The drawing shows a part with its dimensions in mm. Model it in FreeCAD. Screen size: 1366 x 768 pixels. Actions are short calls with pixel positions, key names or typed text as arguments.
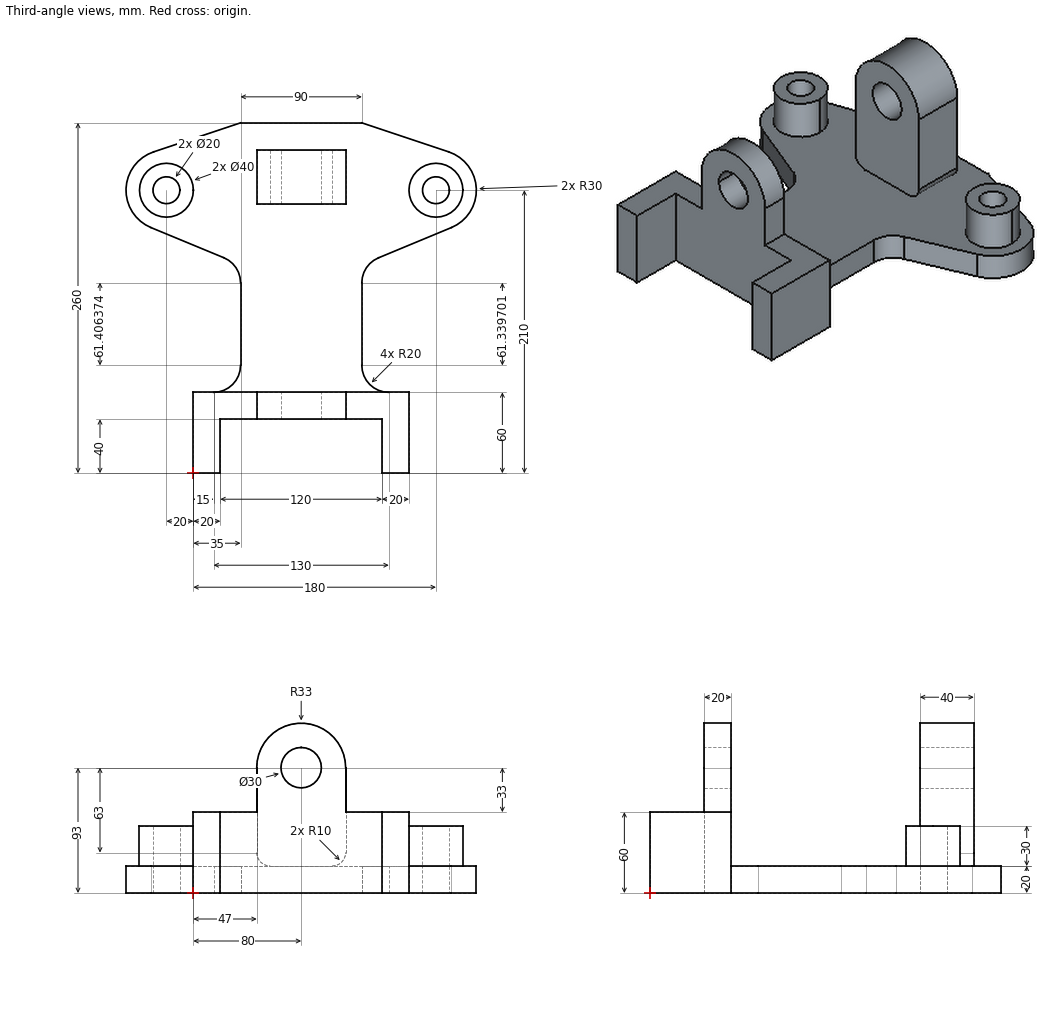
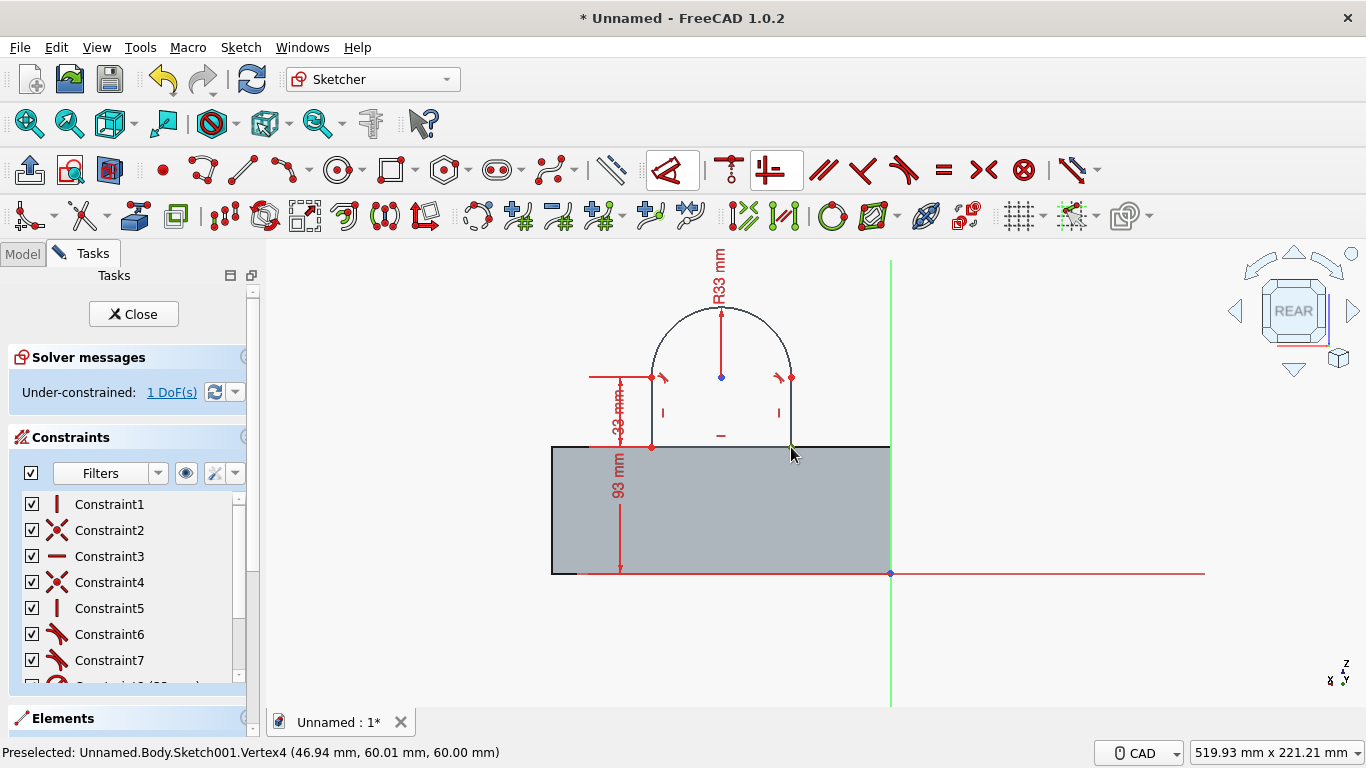
key(l)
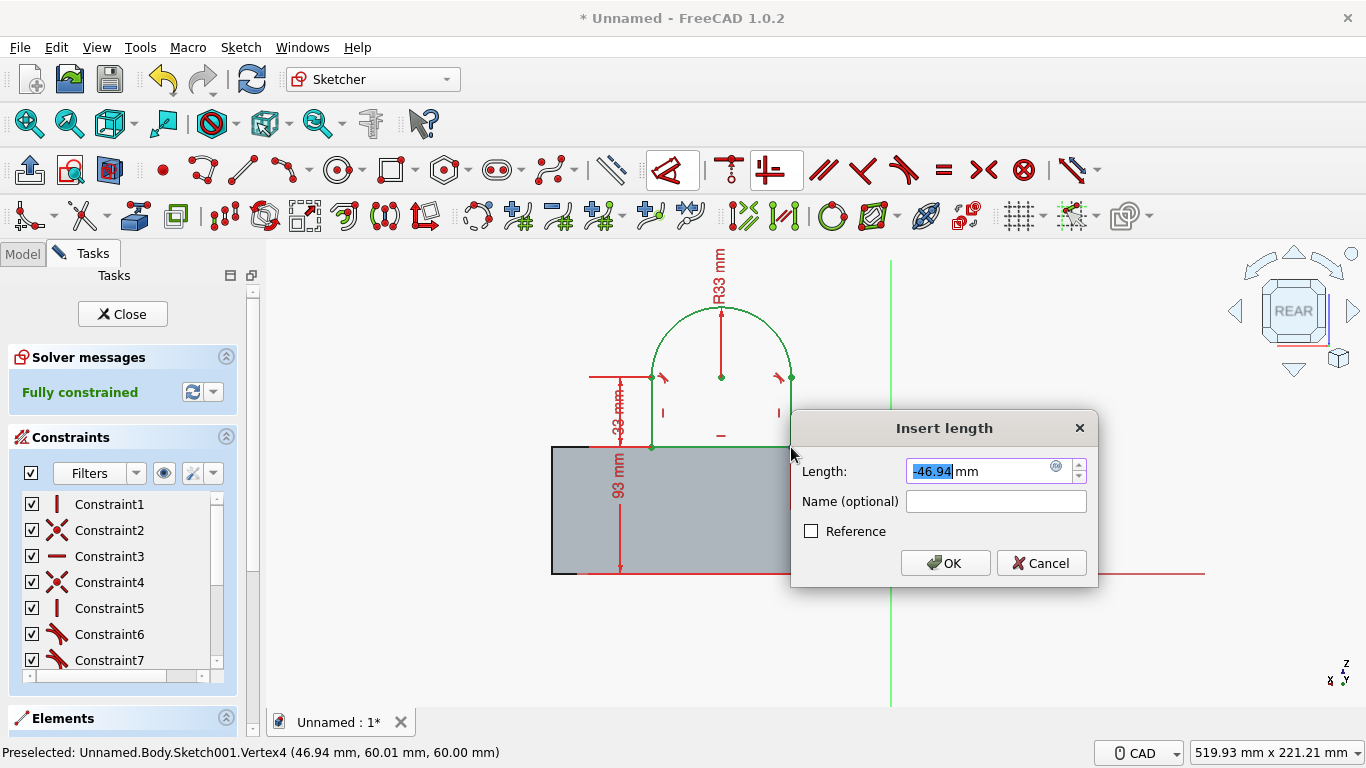
text(-47)
key(Return)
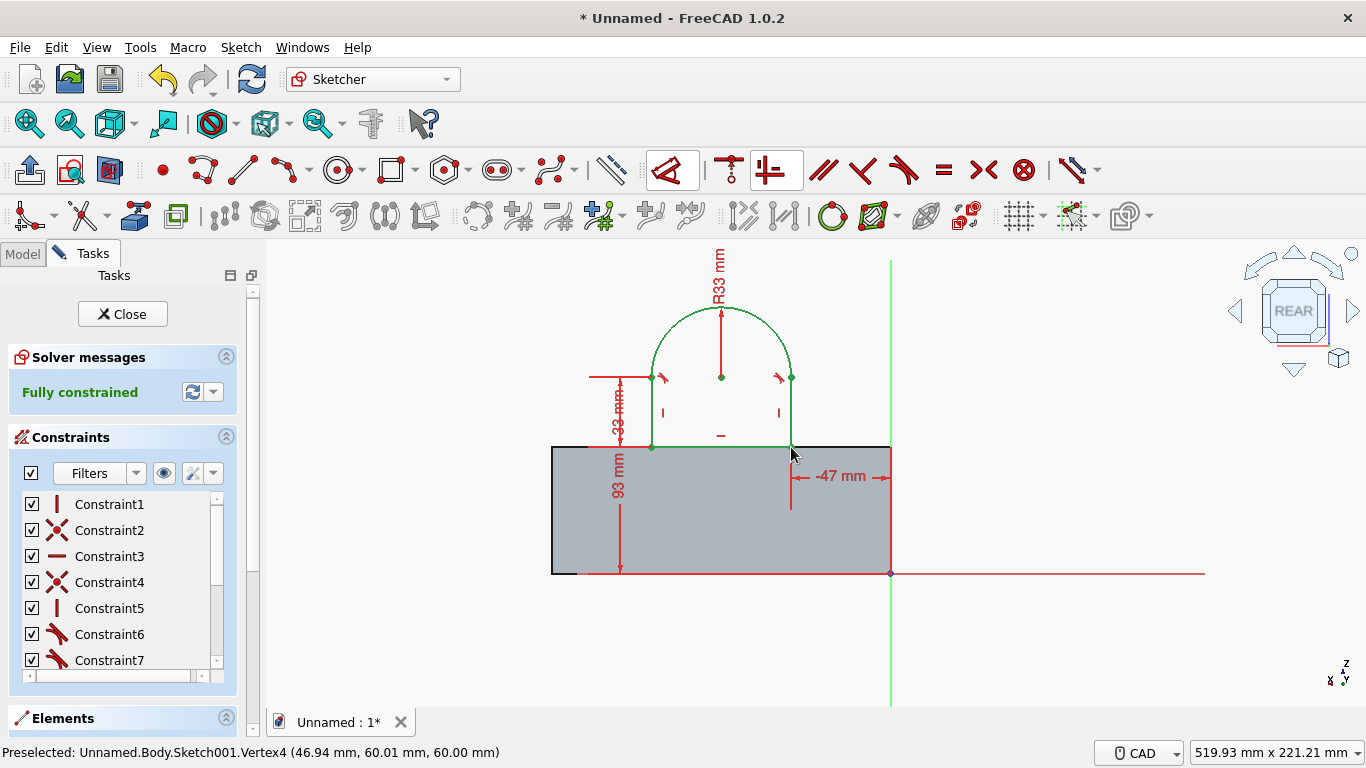
click(123, 314)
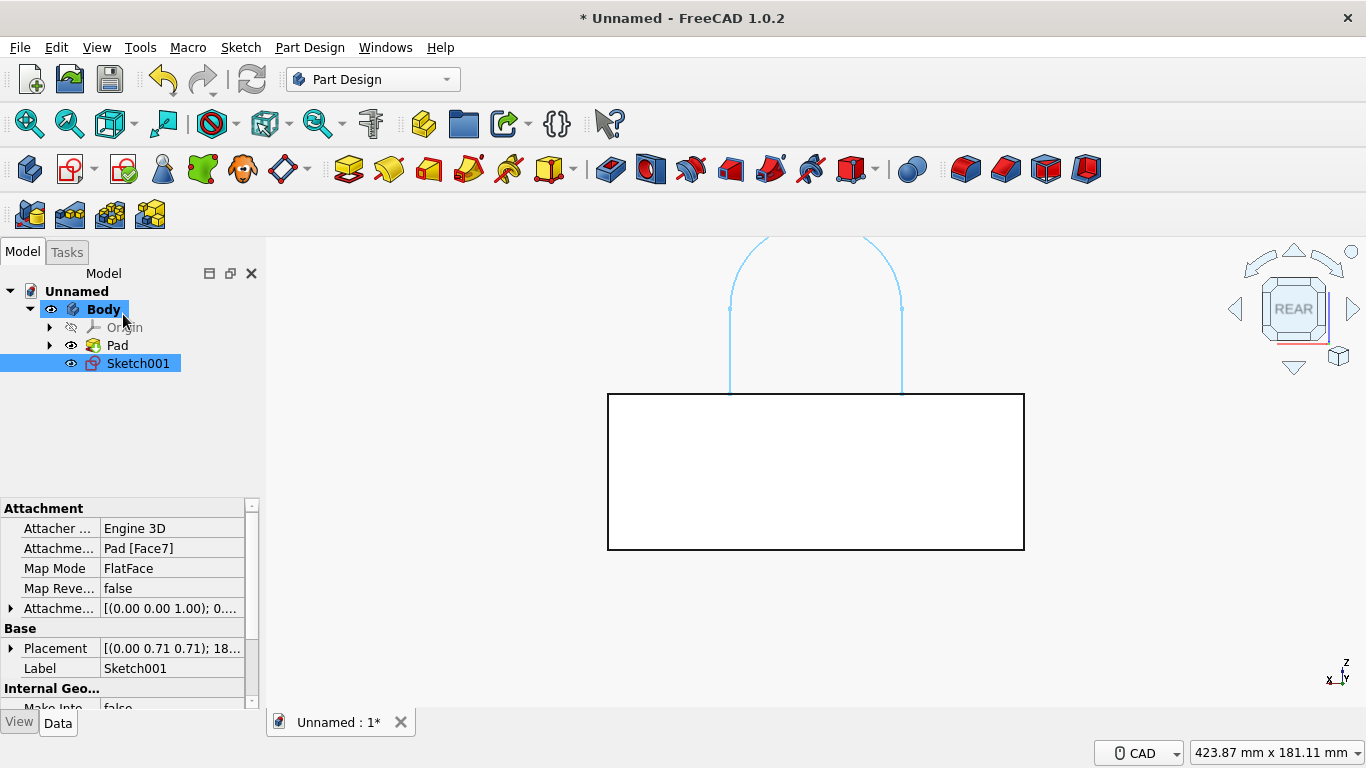
click(350, 170)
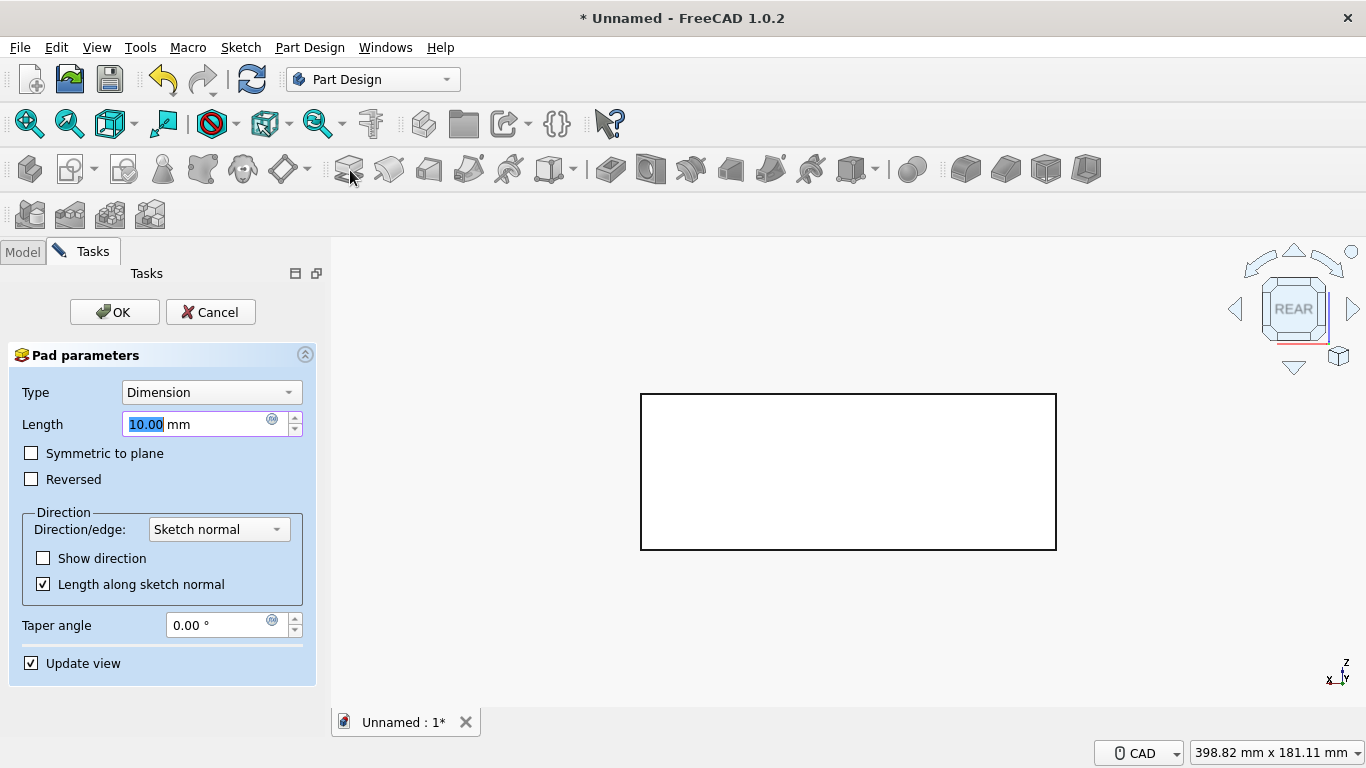
text(20)
key(Tab)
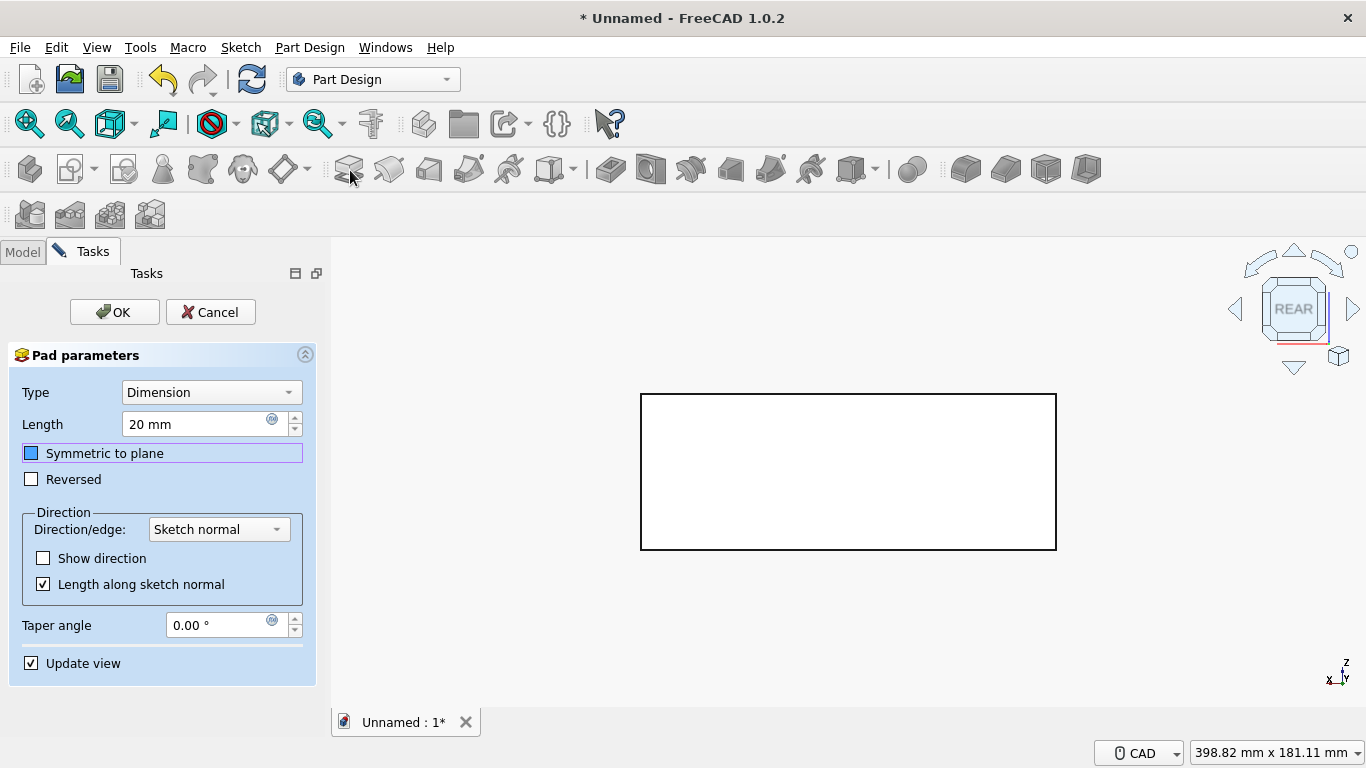
click(30, 479)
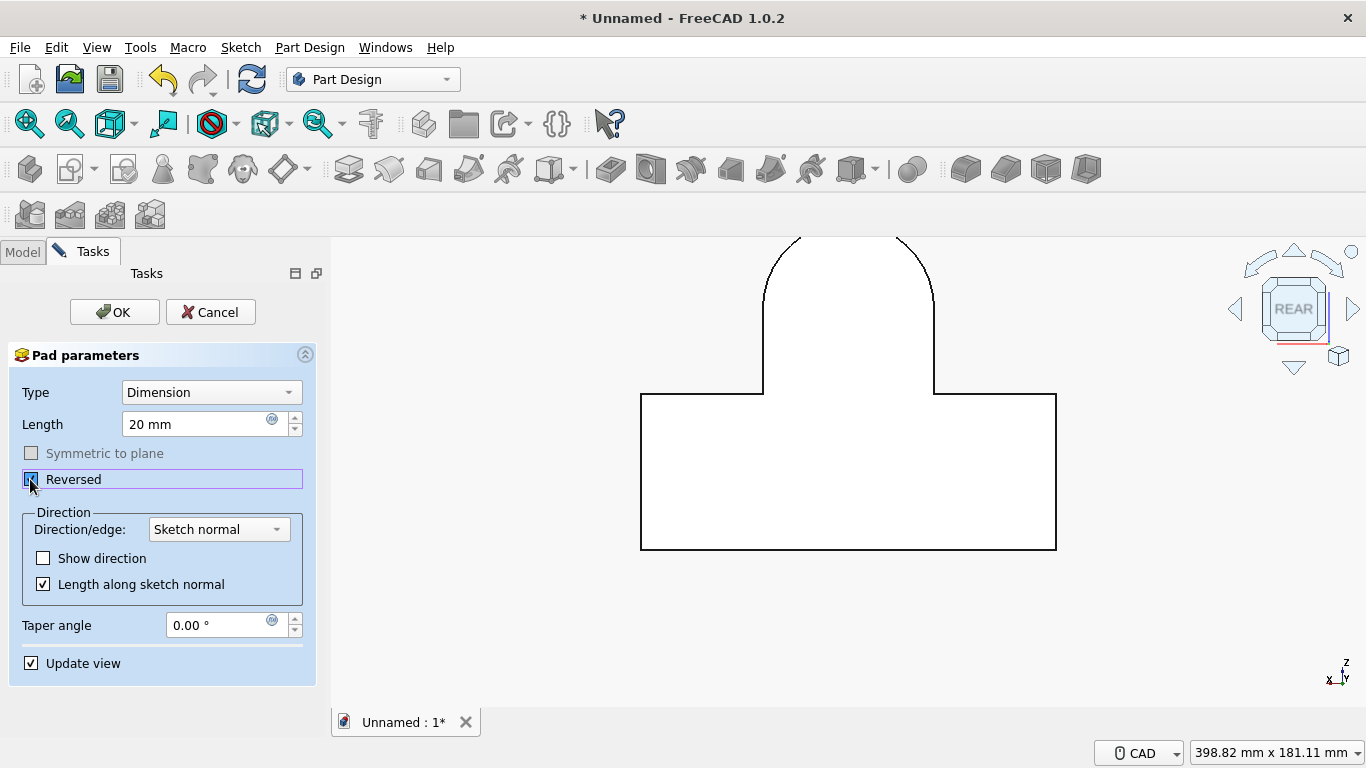
click(115, 312)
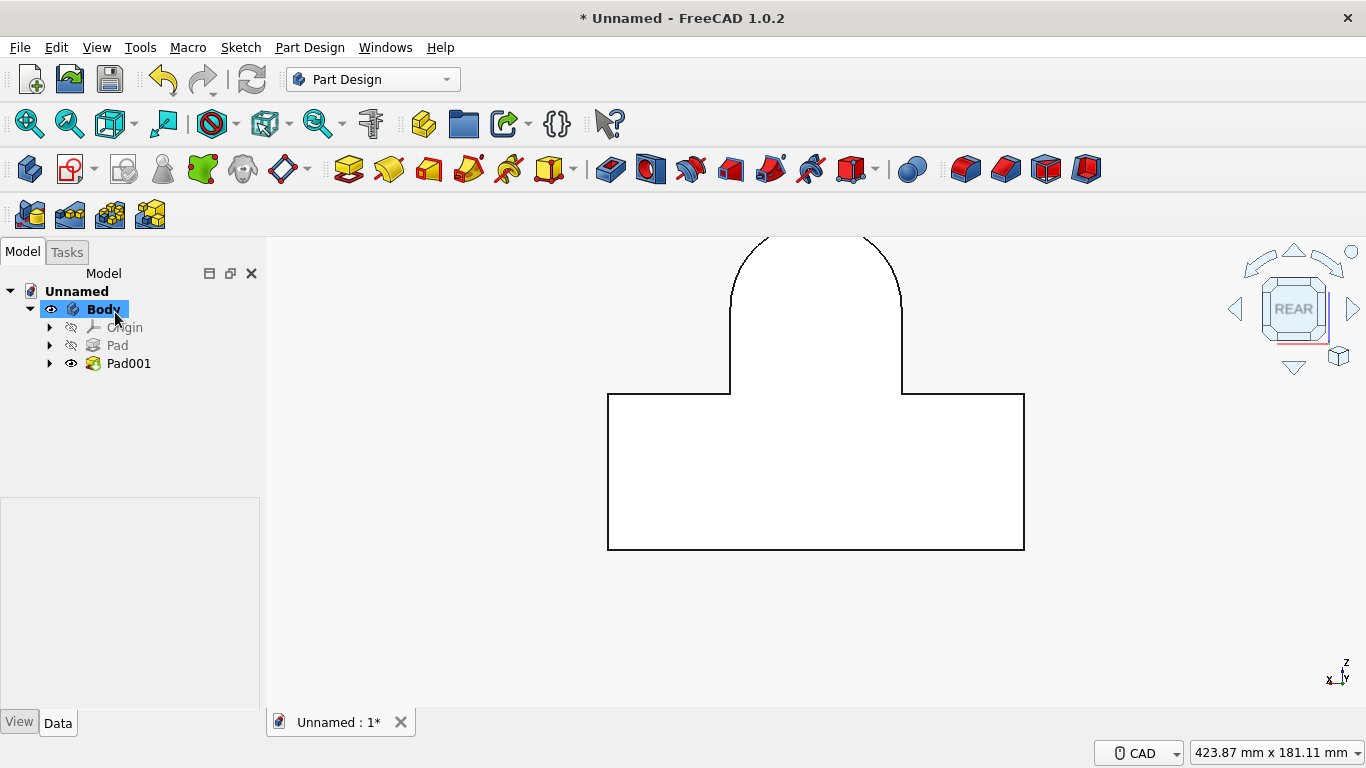
click(30, 124)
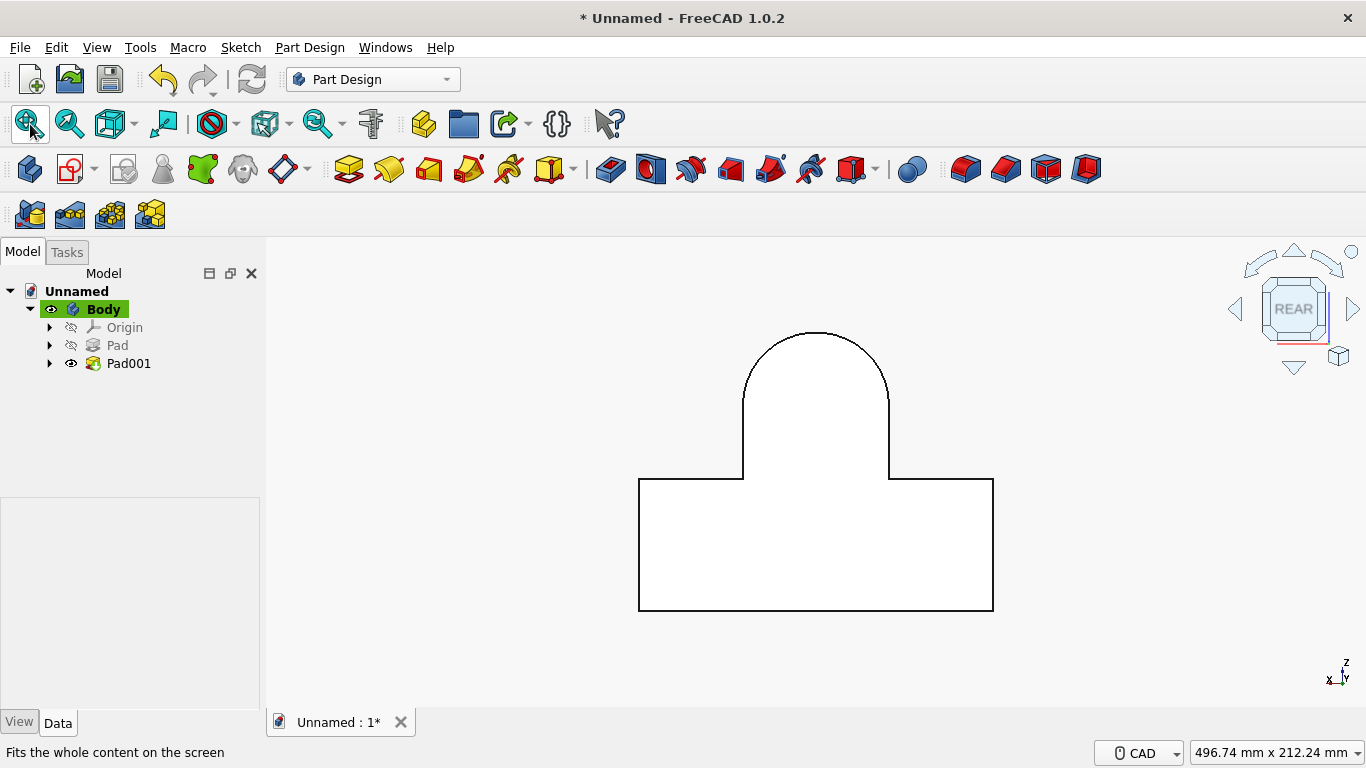
click(816, 511)